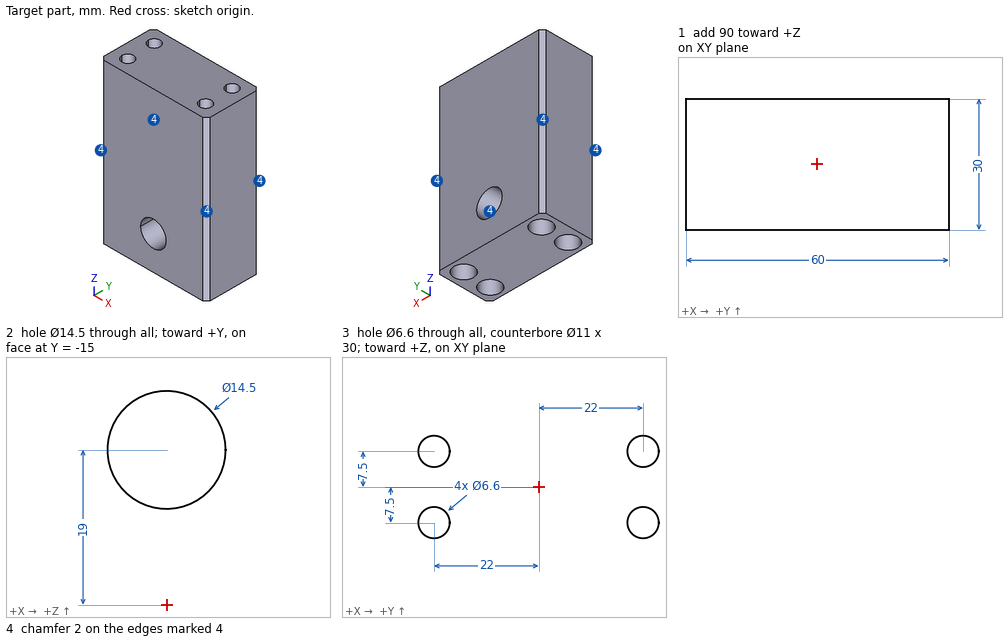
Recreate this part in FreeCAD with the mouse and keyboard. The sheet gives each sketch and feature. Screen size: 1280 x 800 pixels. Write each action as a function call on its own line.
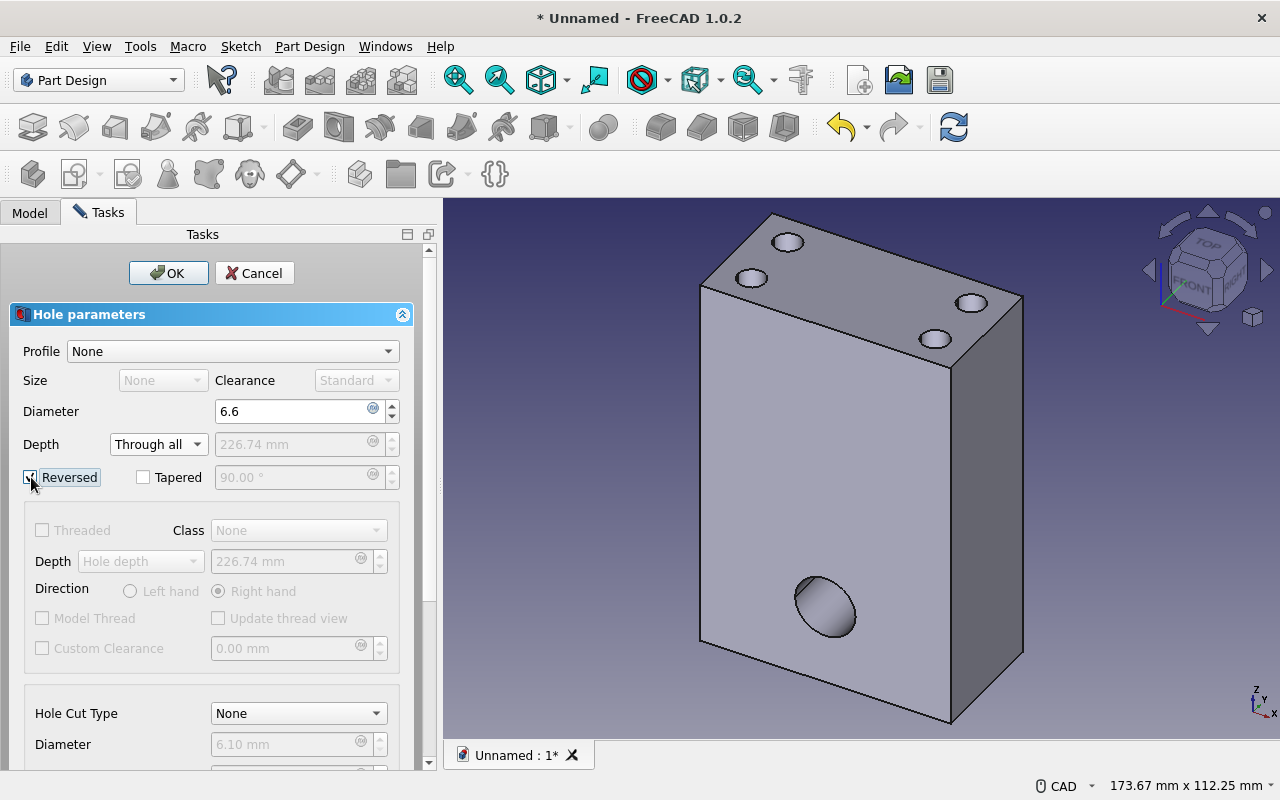
click(300, 714)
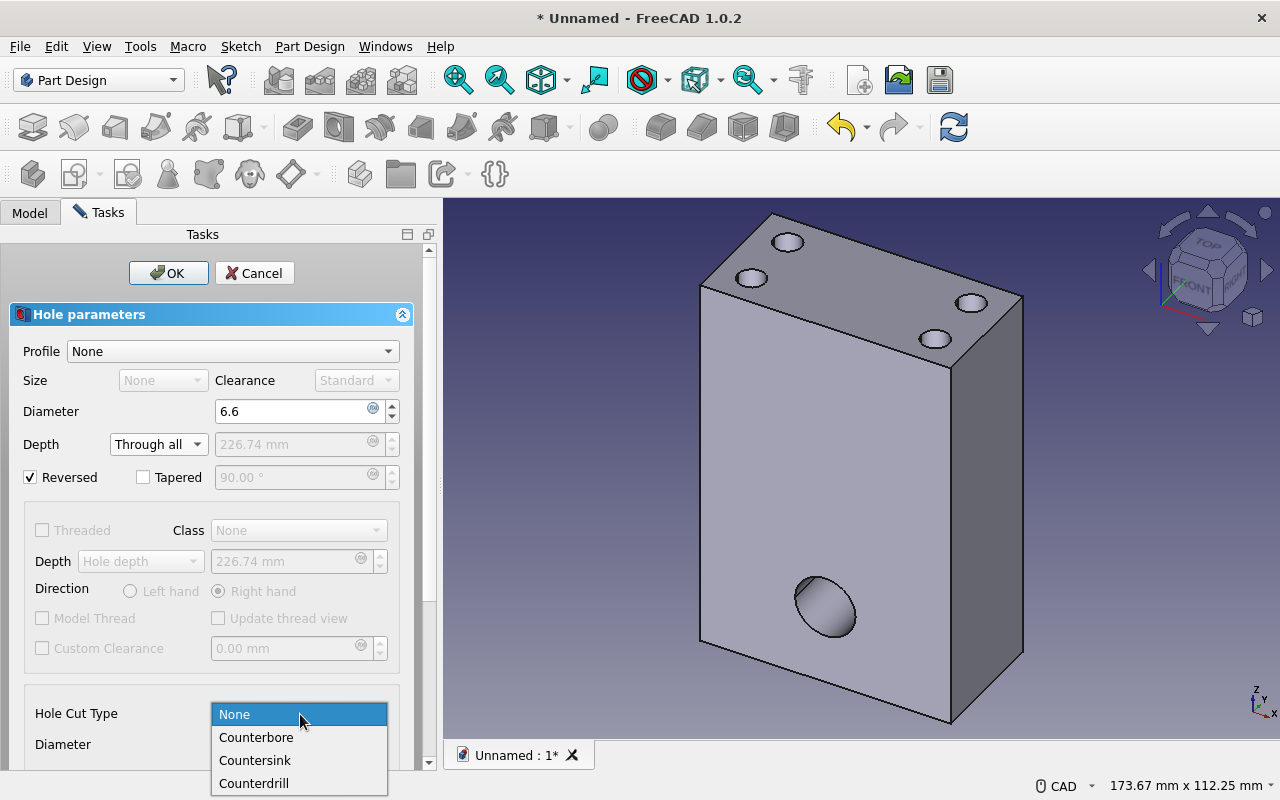
click(298, 738)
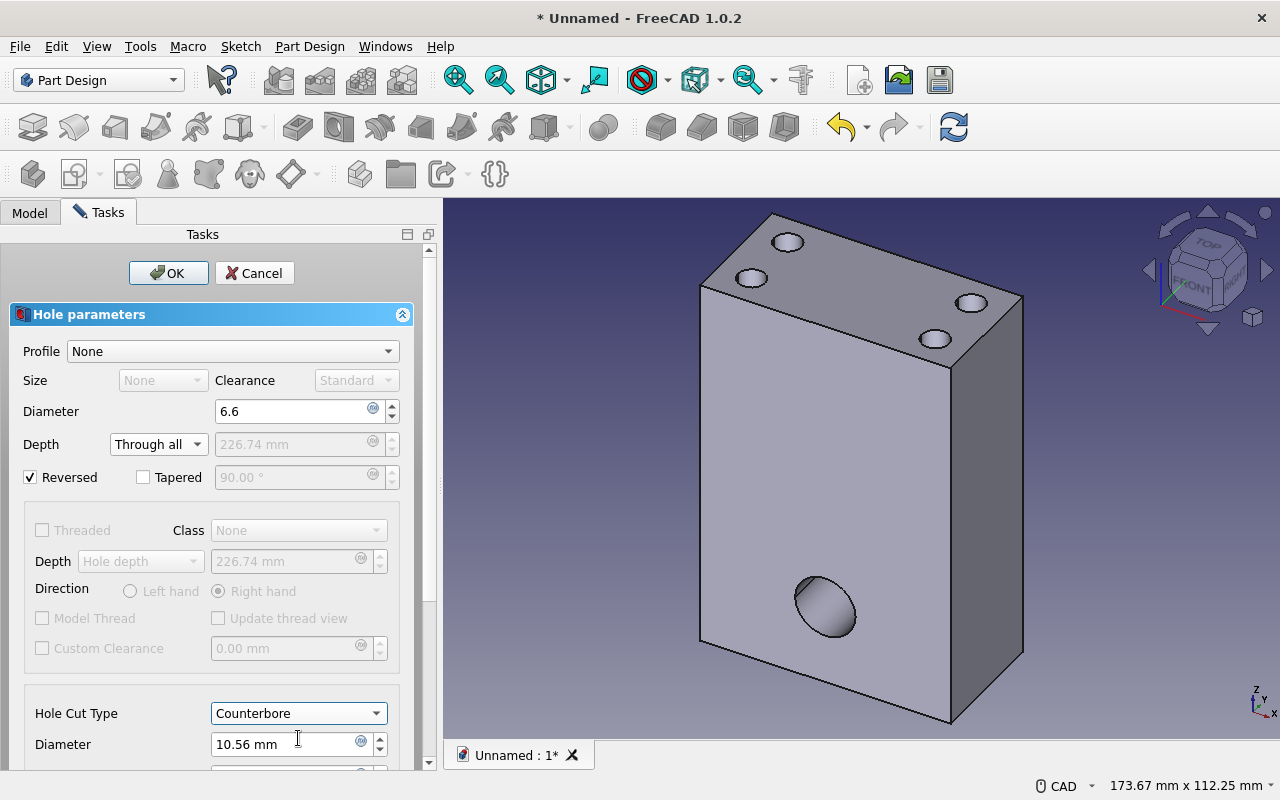
triple_click(292, 744)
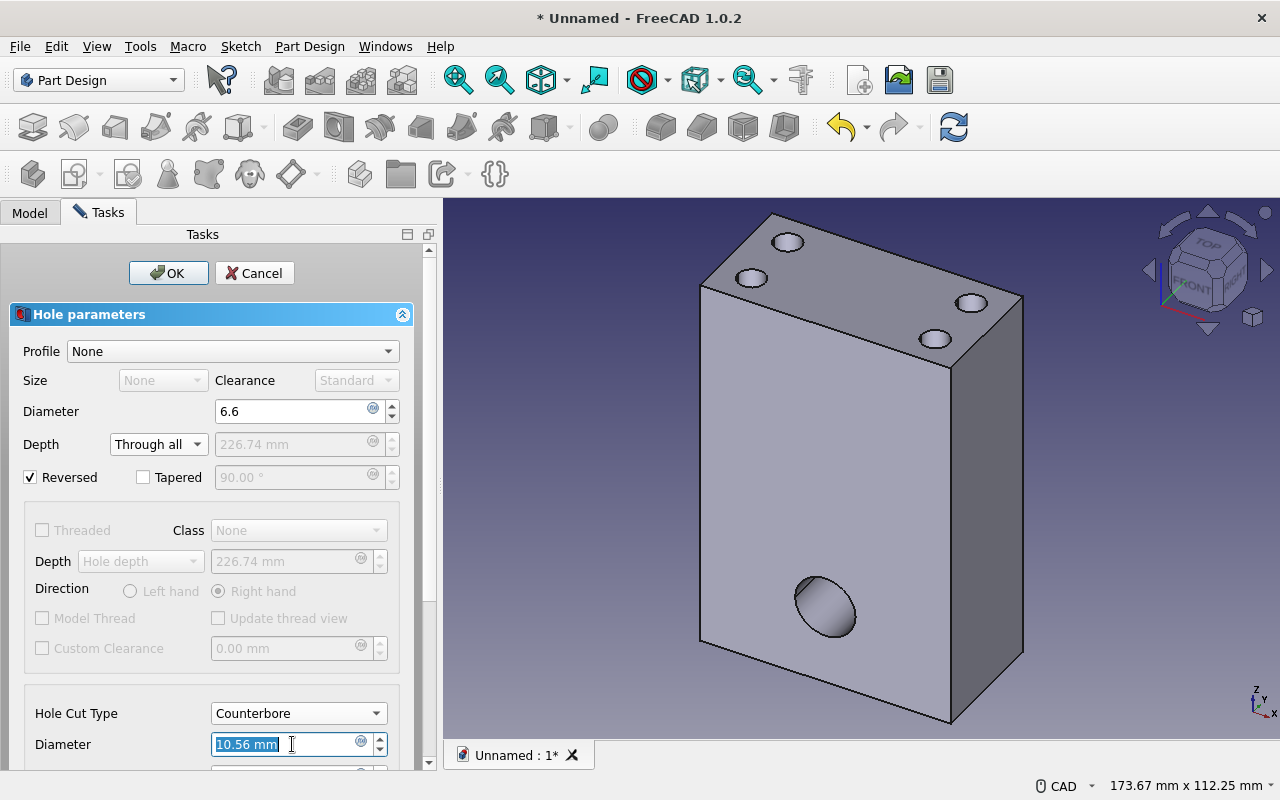
text(11)
key(Tab)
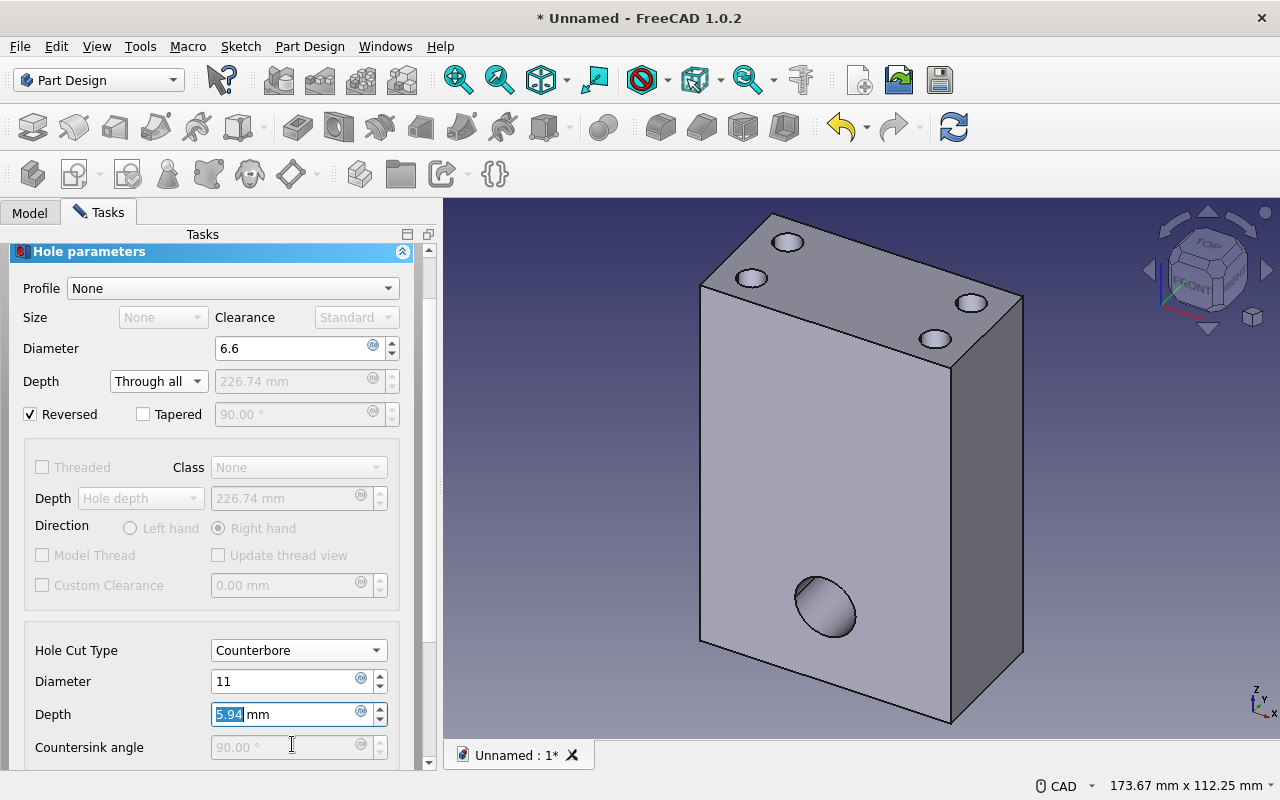
text(30)
key(Tab)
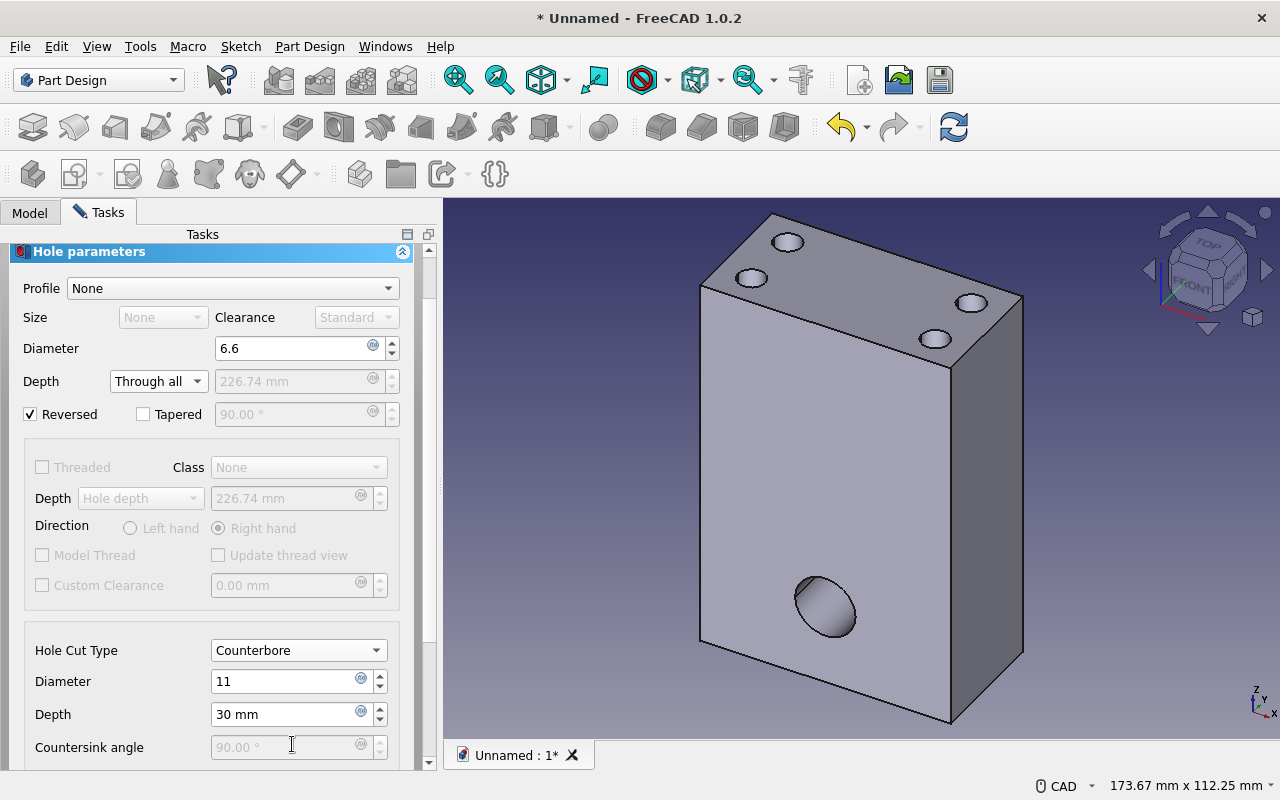
scroll(429, 507, up, 2)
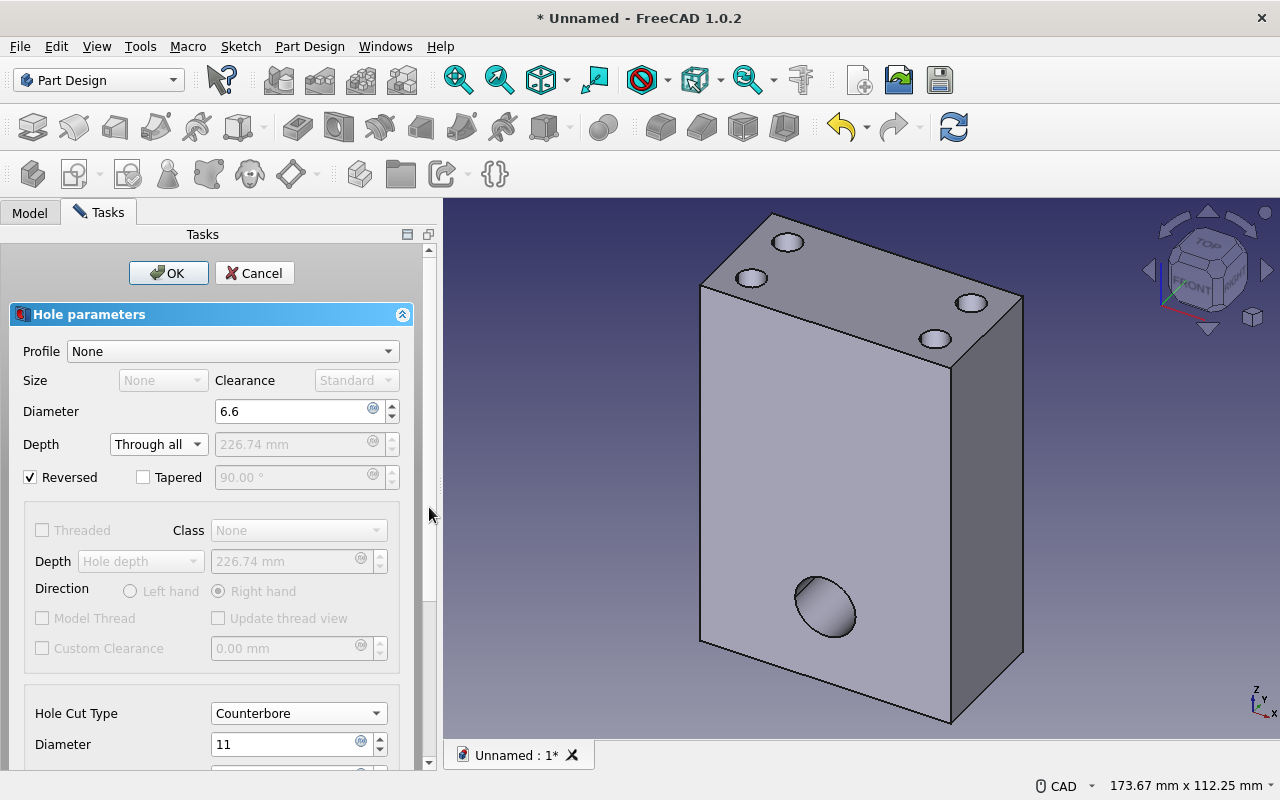
click(169, 273)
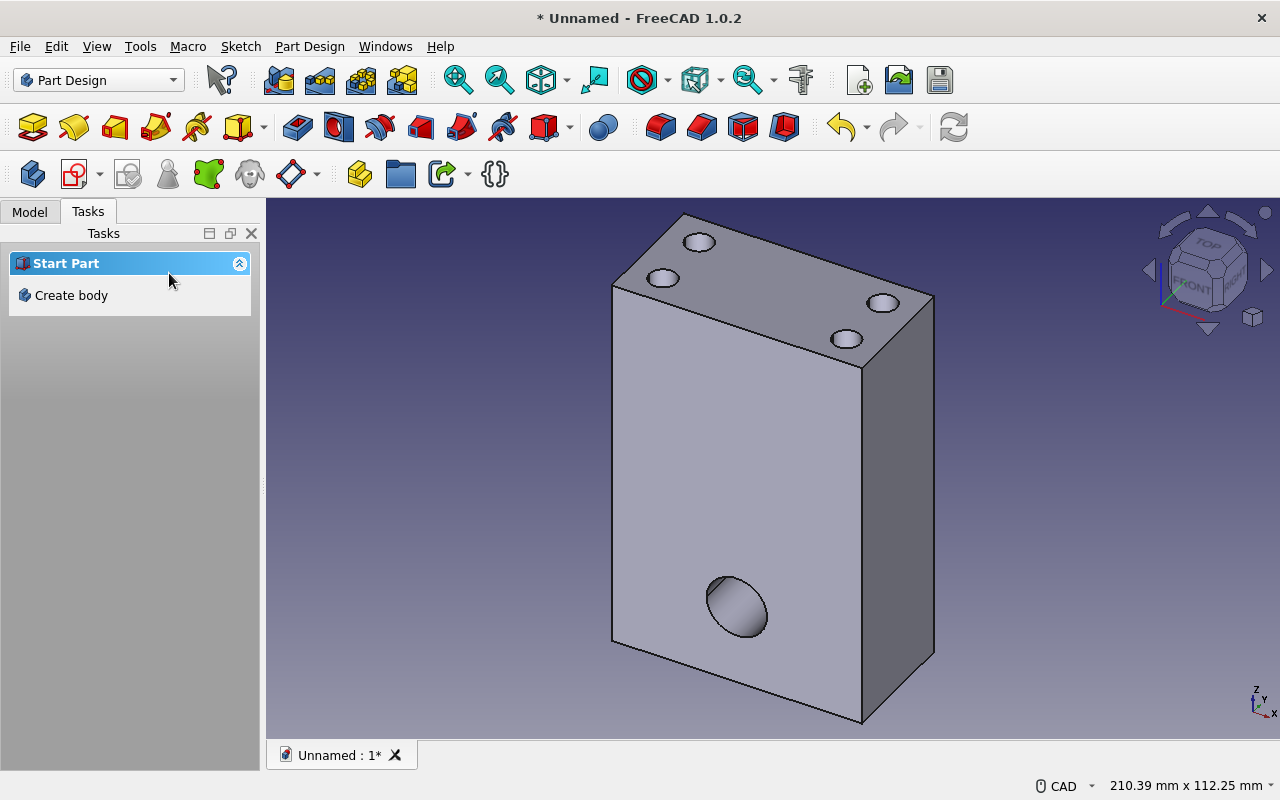
click(862, 545)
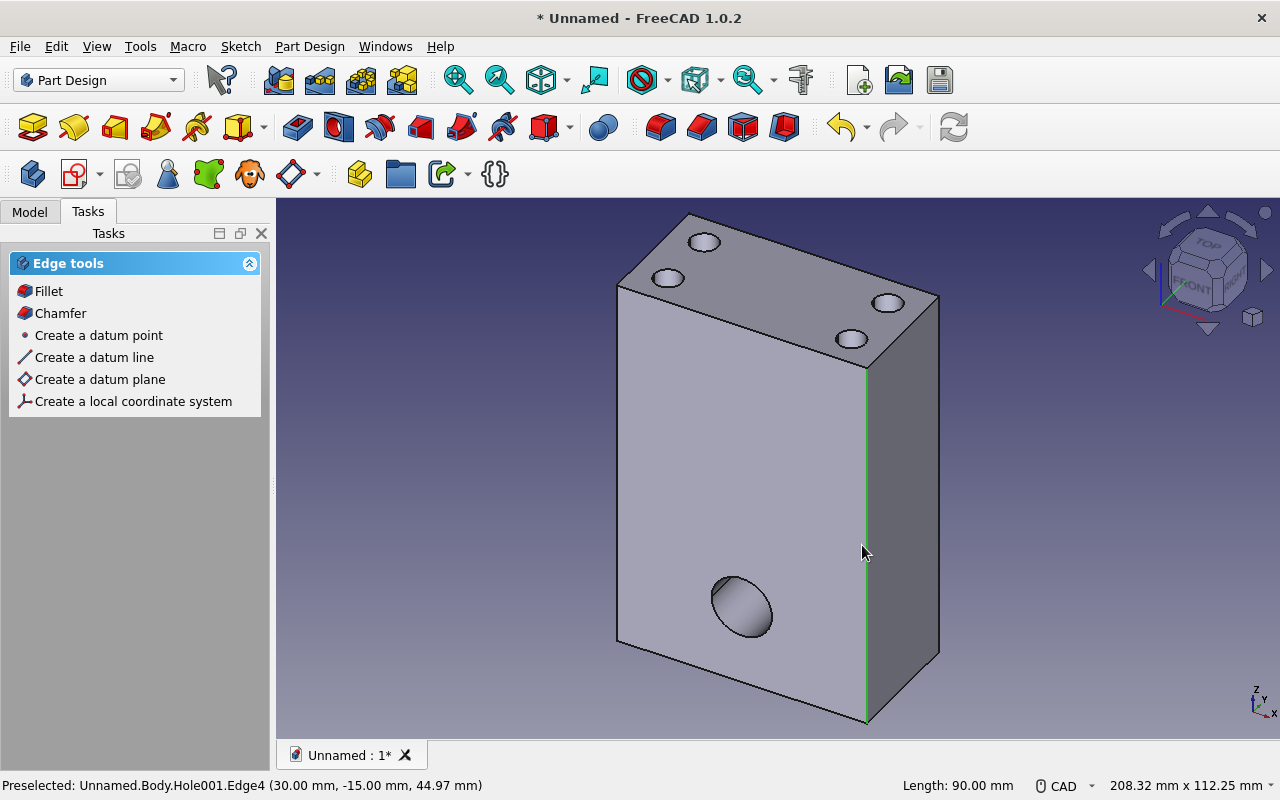
key(0)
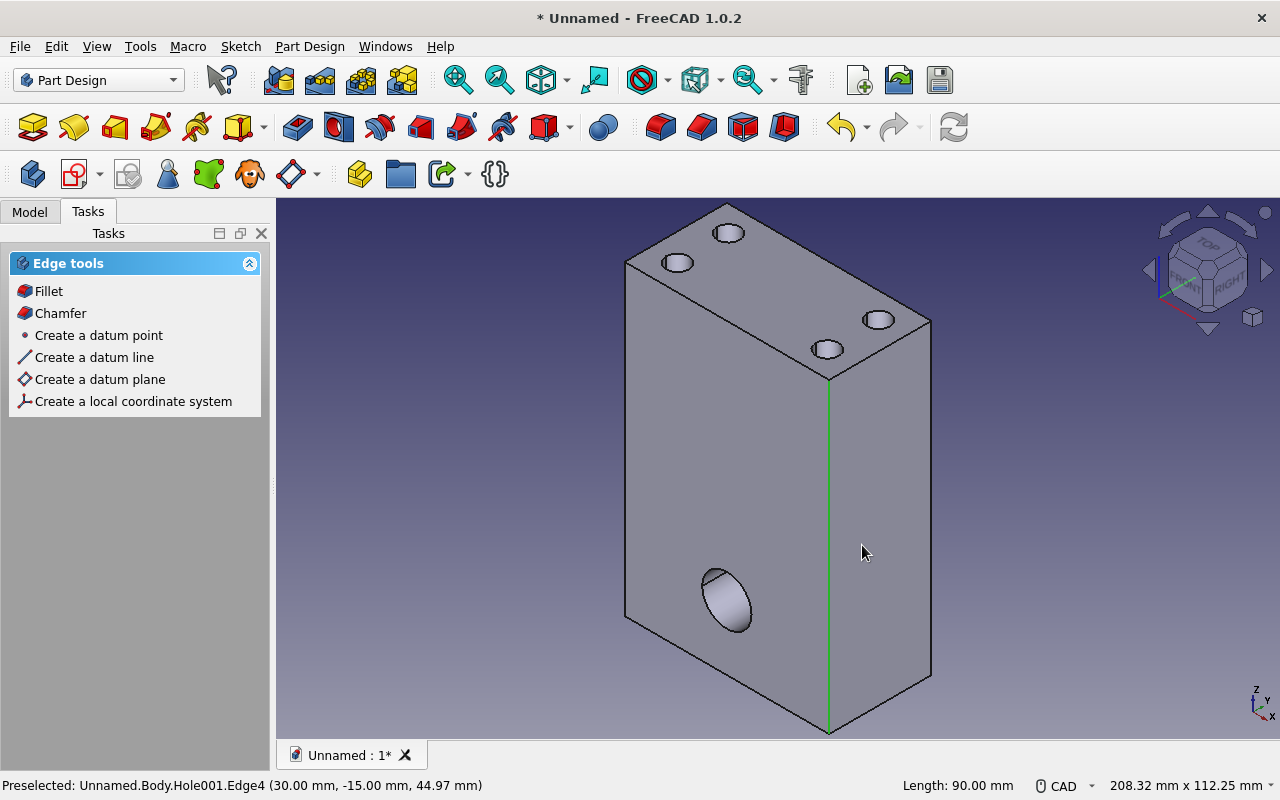
key(2)